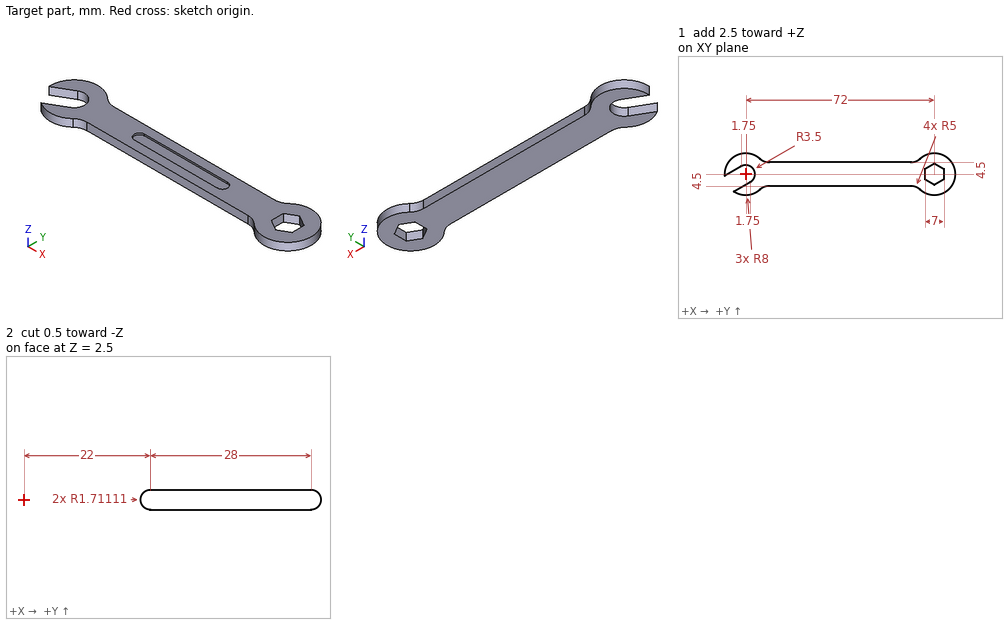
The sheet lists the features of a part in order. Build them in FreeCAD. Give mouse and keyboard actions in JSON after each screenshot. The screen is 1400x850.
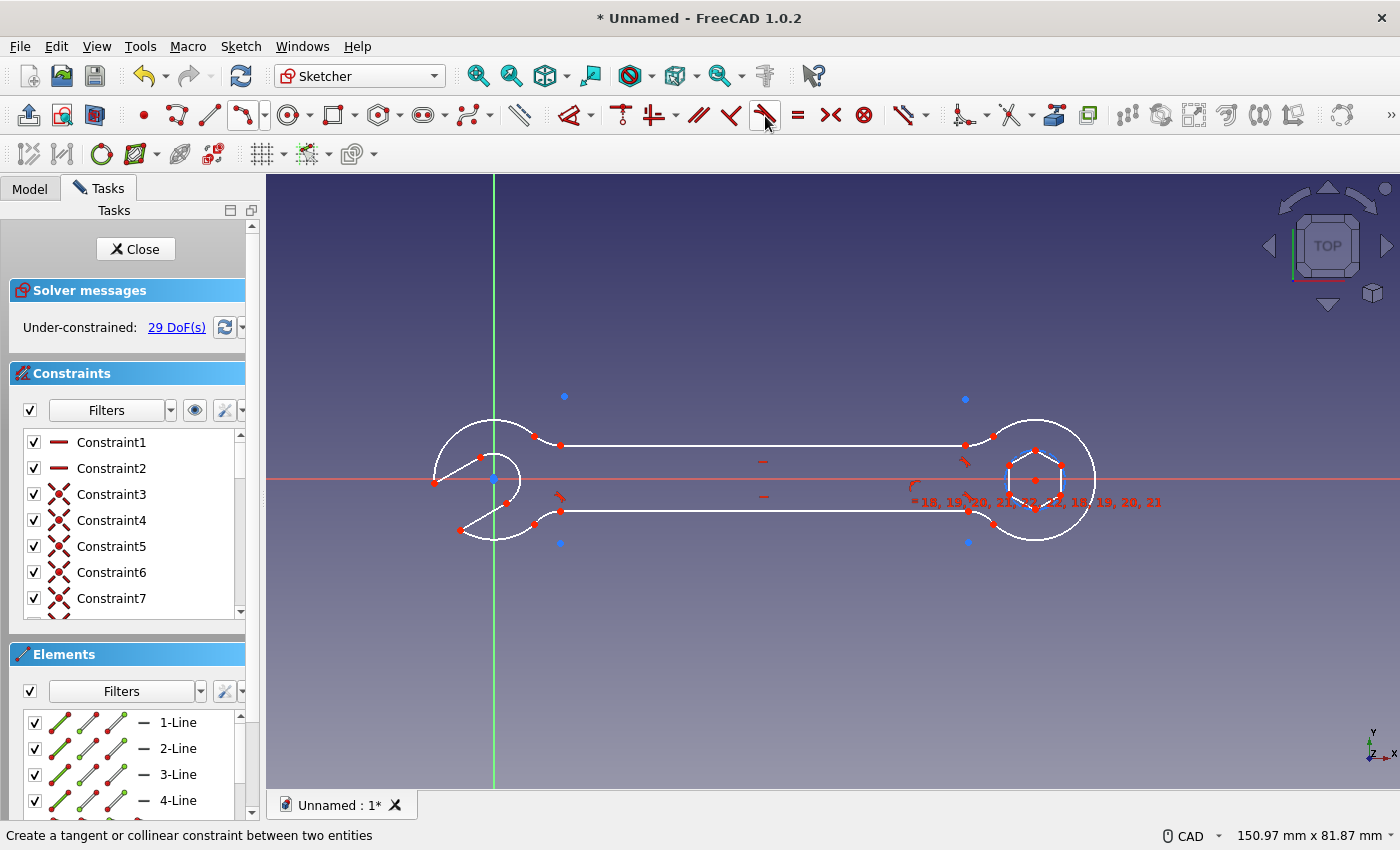
{"action": "left_click", "coordinate": [844, 446]}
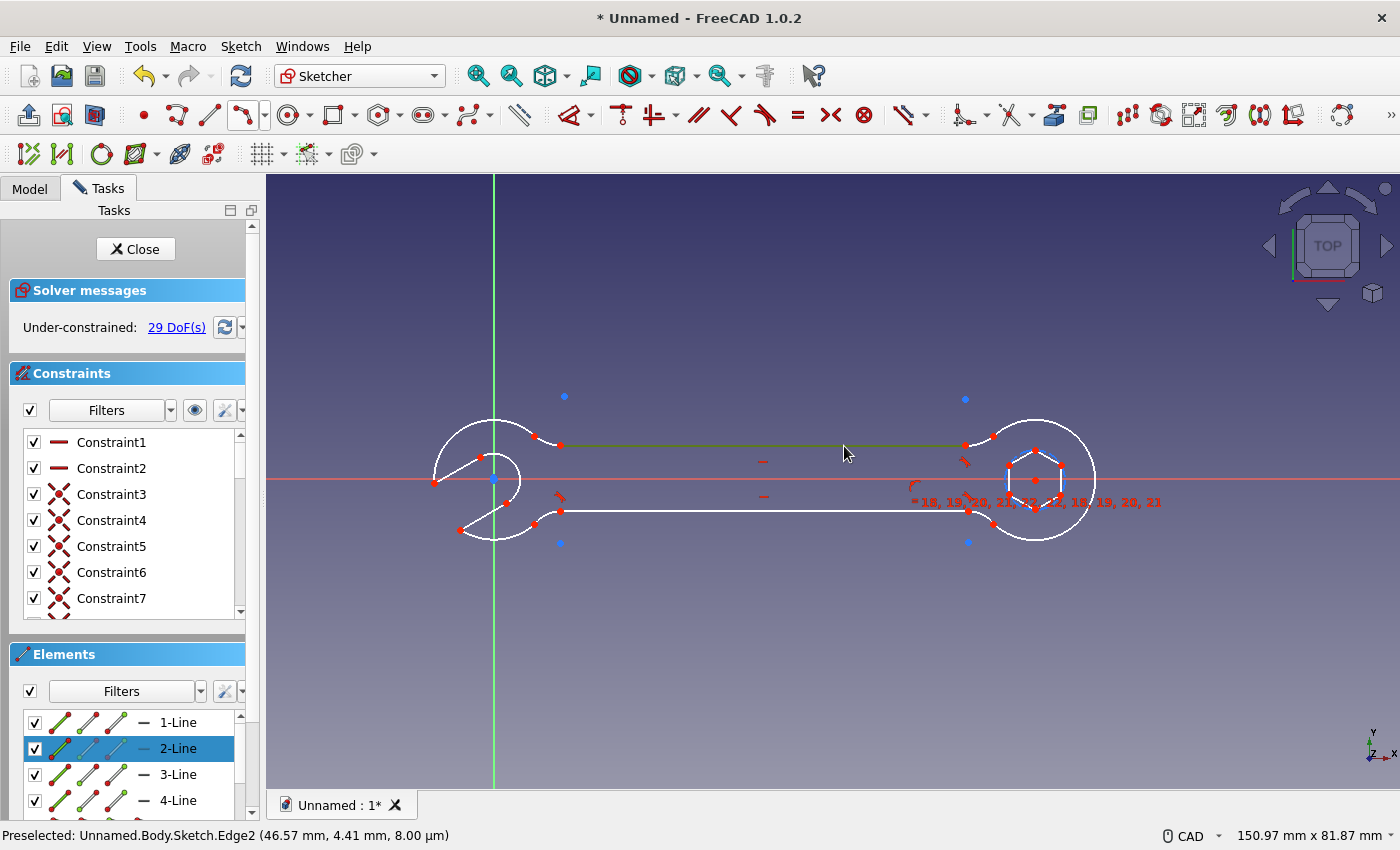
{"action": "left_click", "coordinate": [547, 443]}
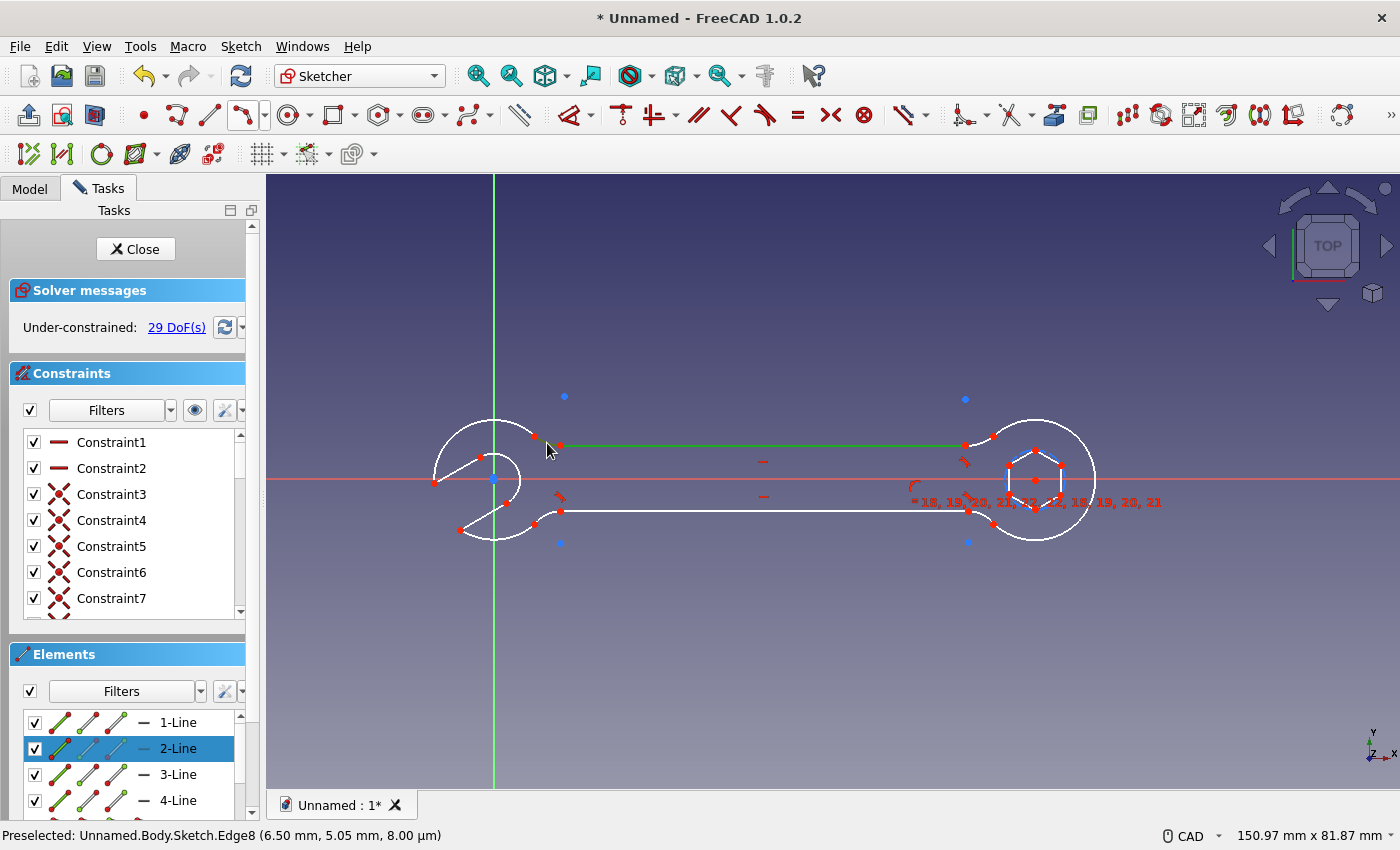
{"action": "key", "text": "t"}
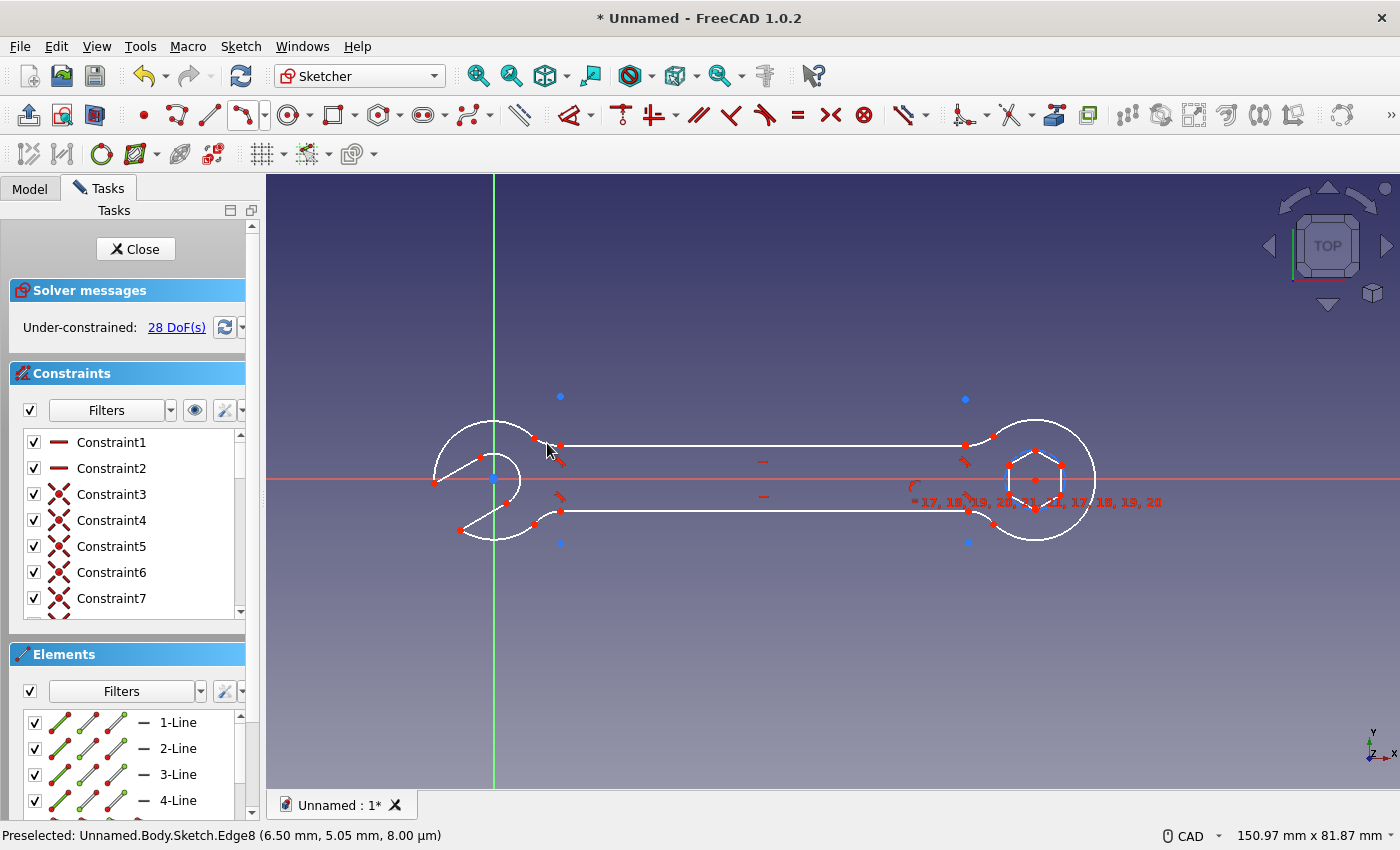
{"action": "left_click", "coordinate": [448, 476]}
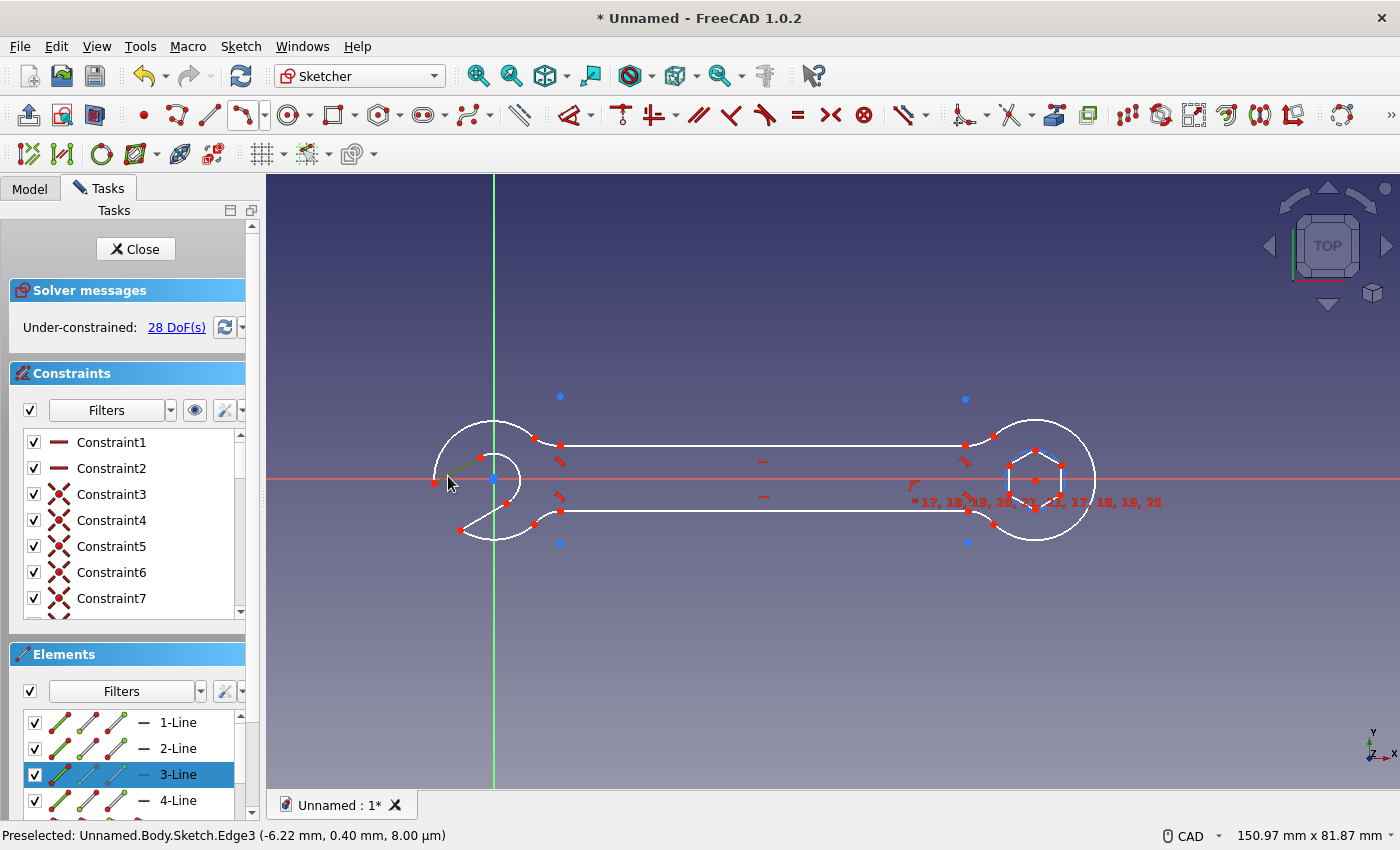
{"action": "left_click", "coordinate": [520, 483]}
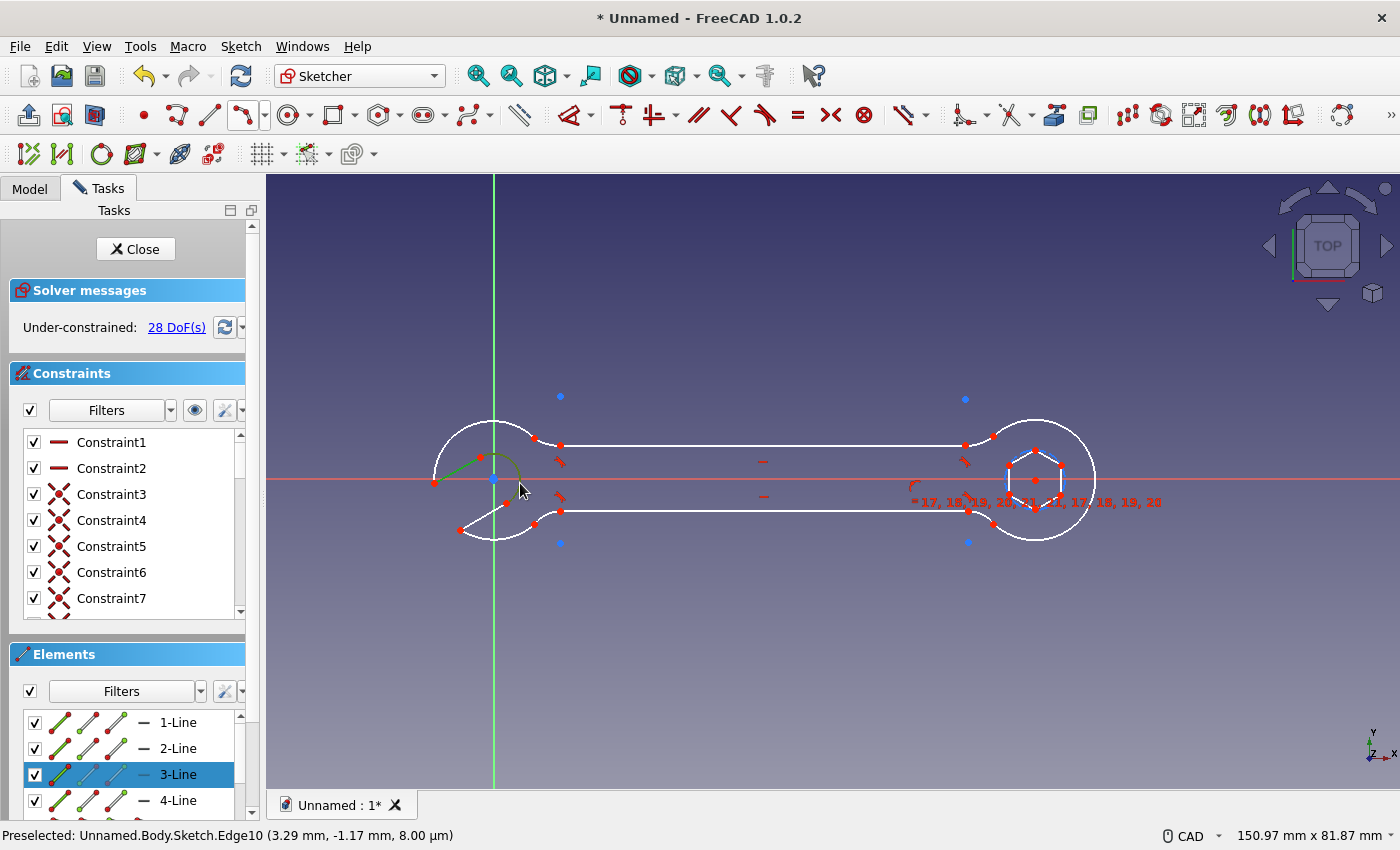
{"action": "left_click", "coordinate": [765, 116]}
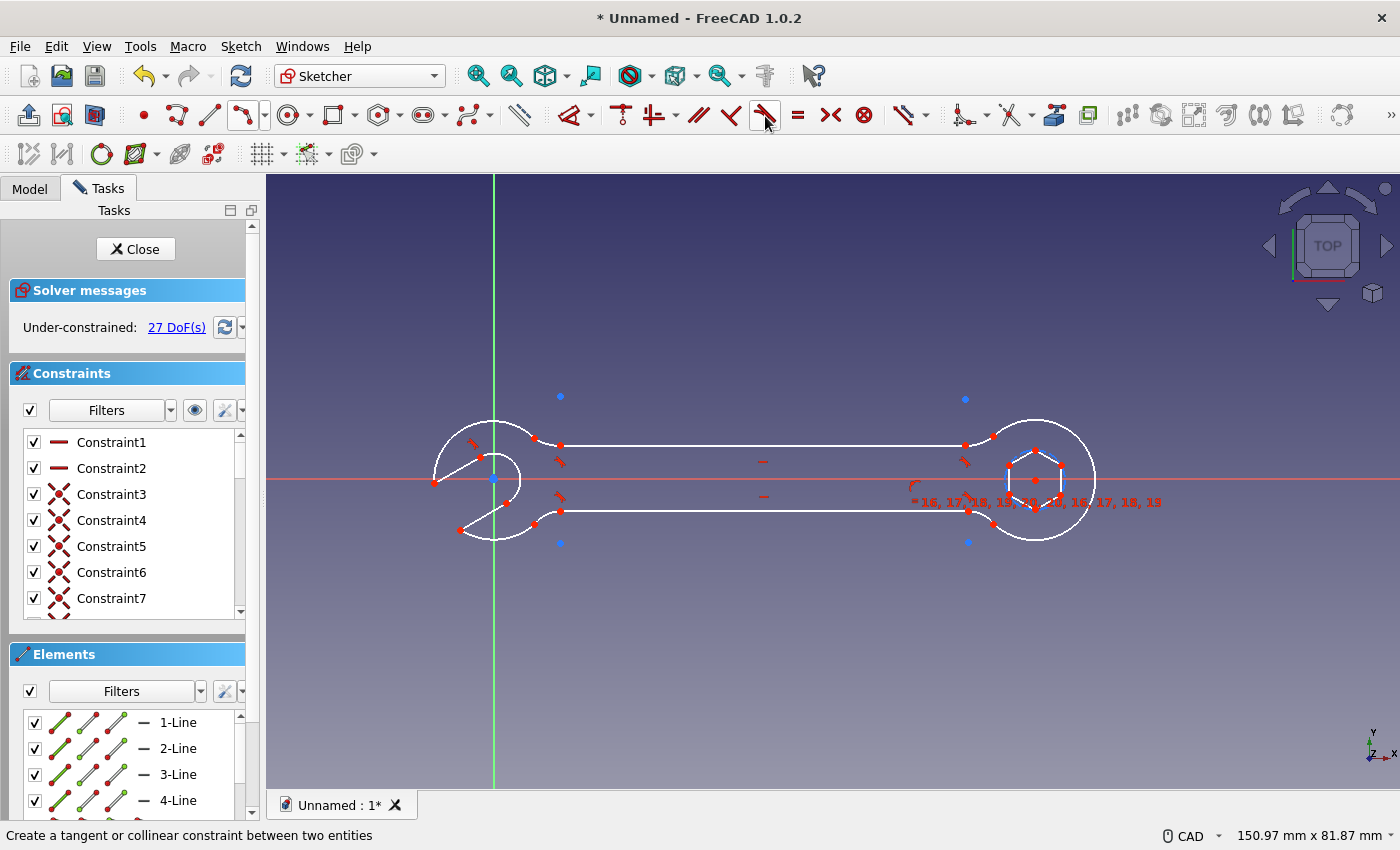
{"action": "left_click", "coordinate": [493, 511]}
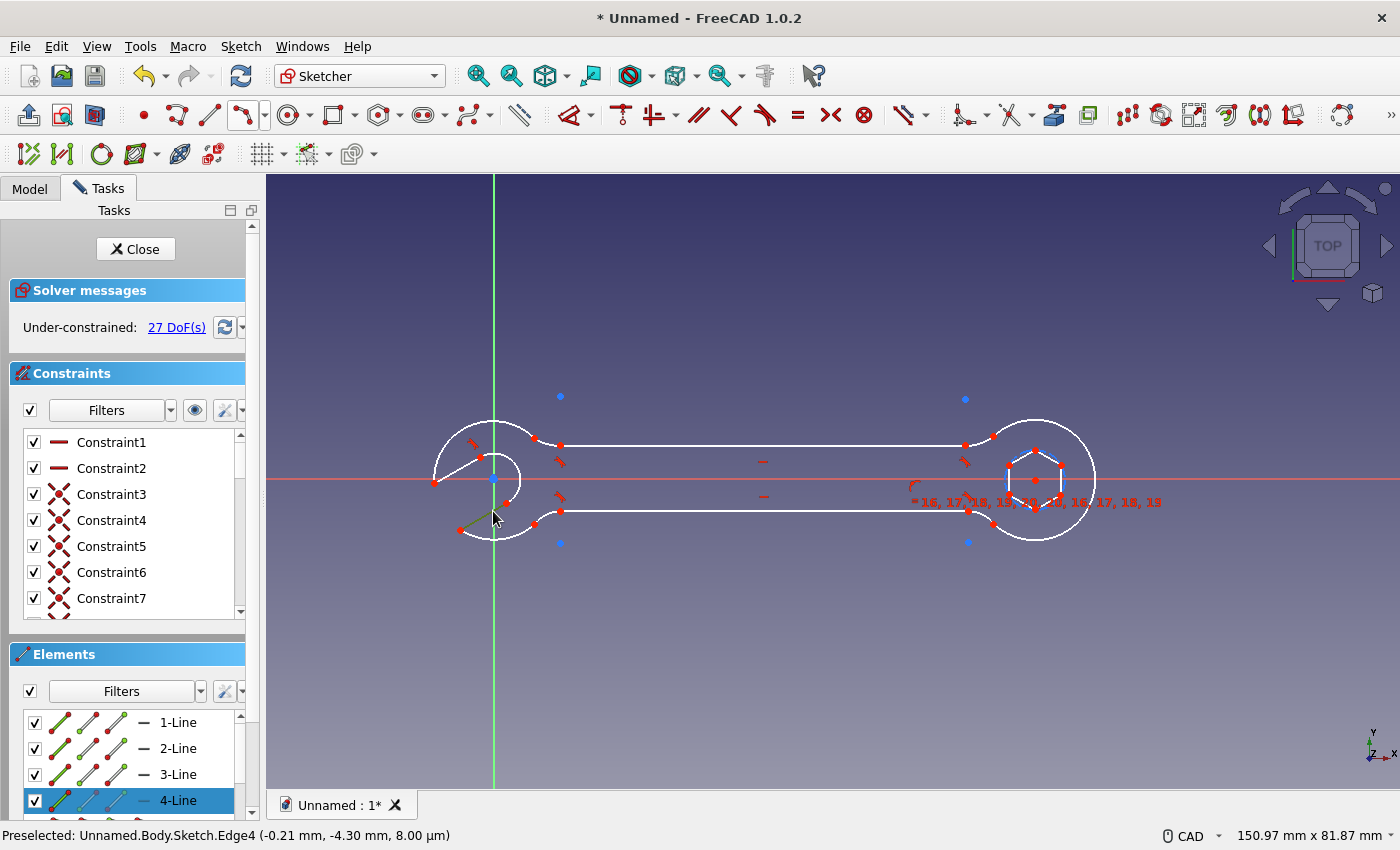
{"action": "left_click", "coordinate": [520, 483]}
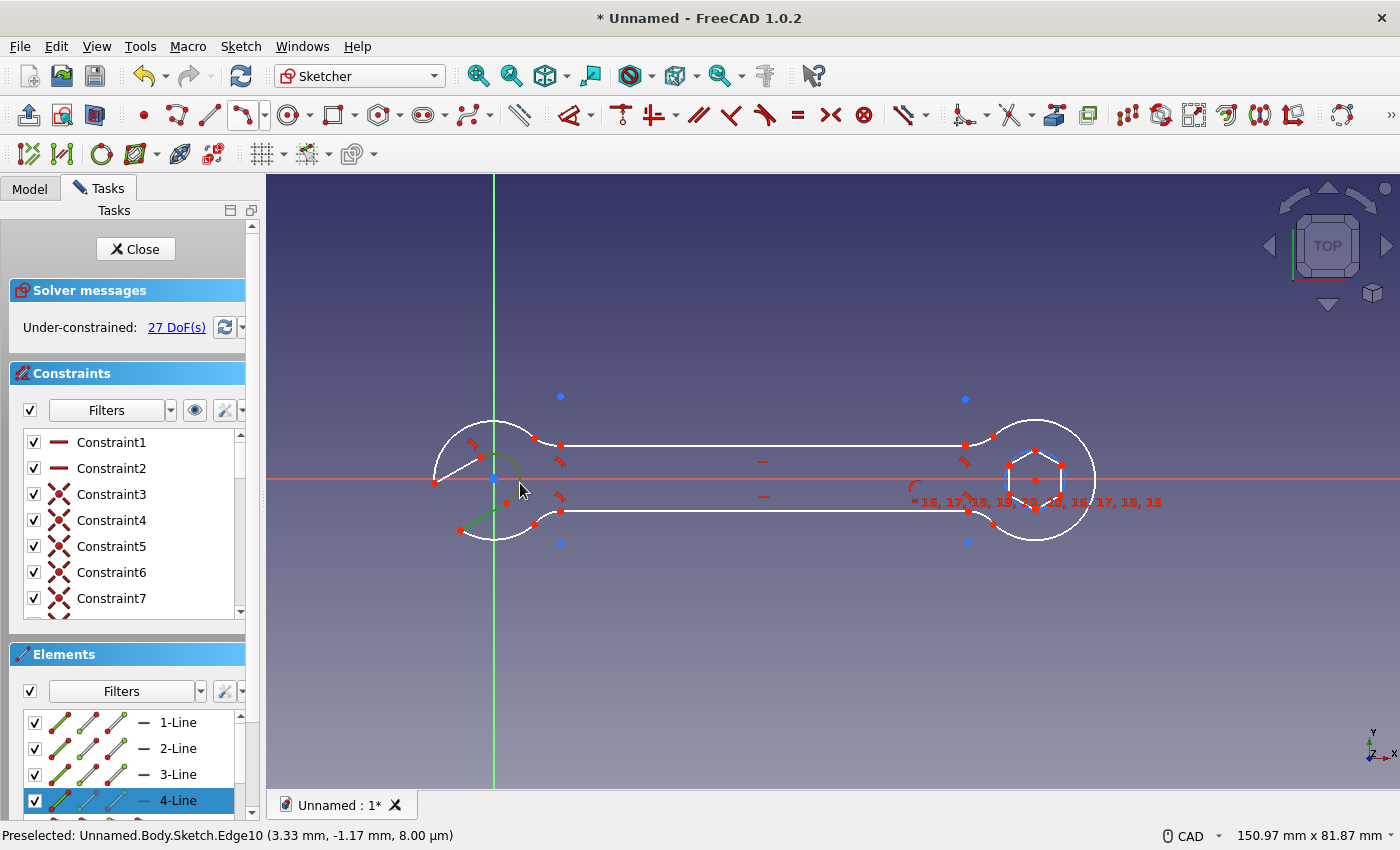
{"action": "key", "text": "t"}